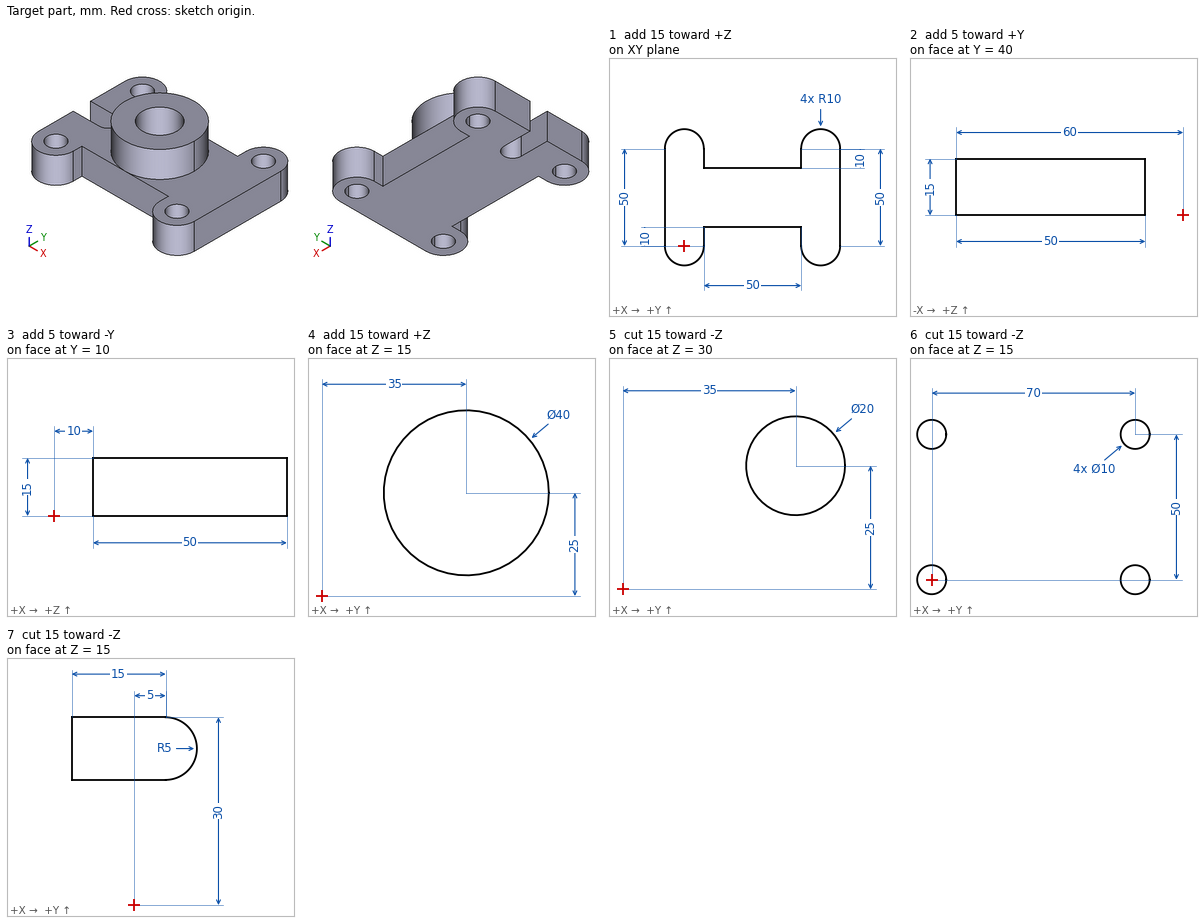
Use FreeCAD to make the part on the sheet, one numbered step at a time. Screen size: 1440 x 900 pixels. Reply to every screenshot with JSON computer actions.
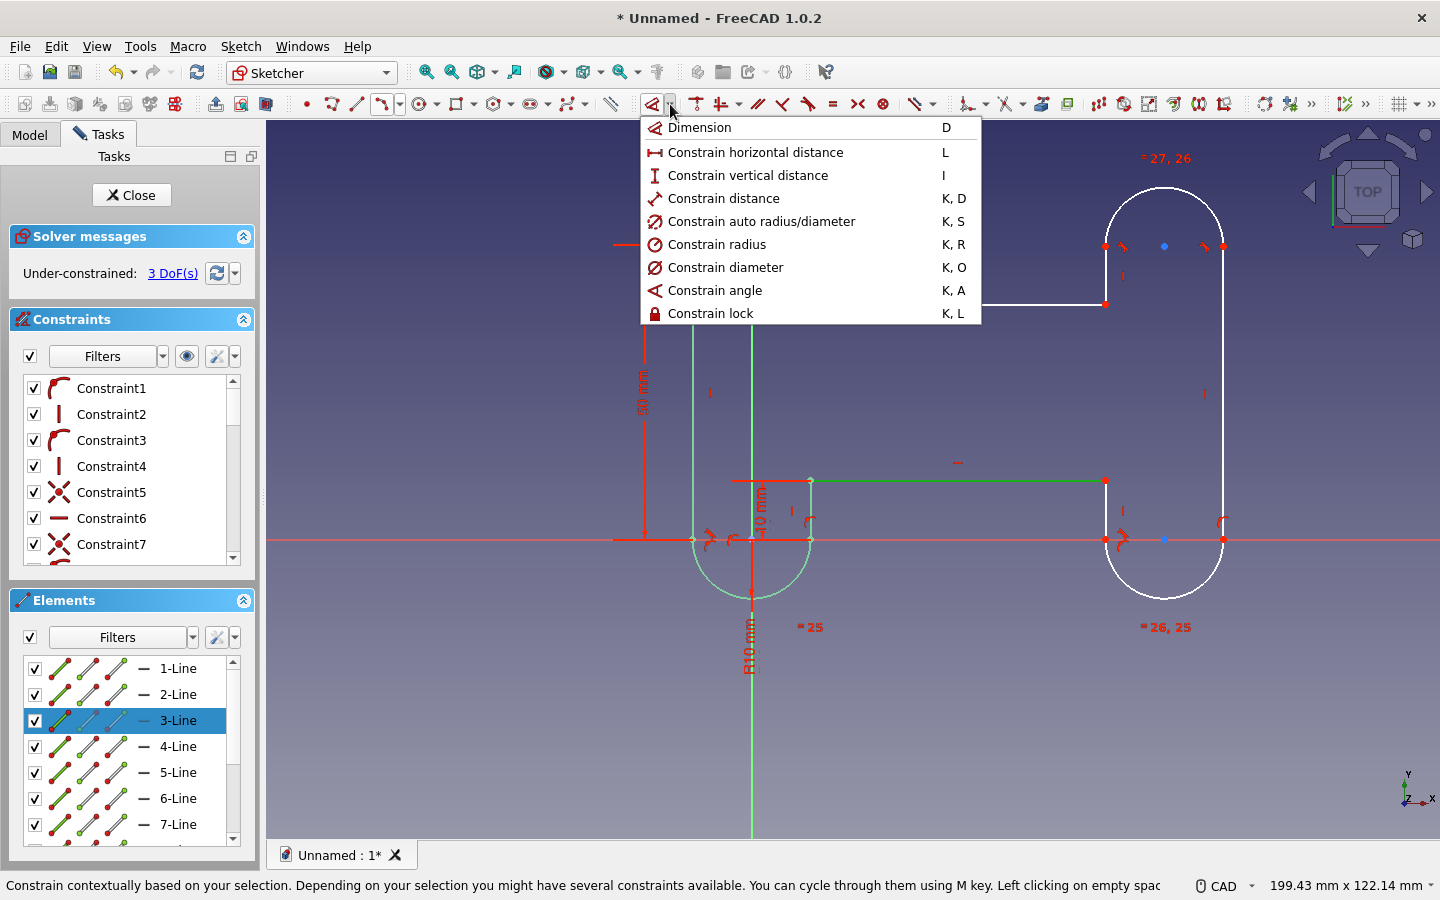
{"action": "left_click", "coordinate": [811, 152]}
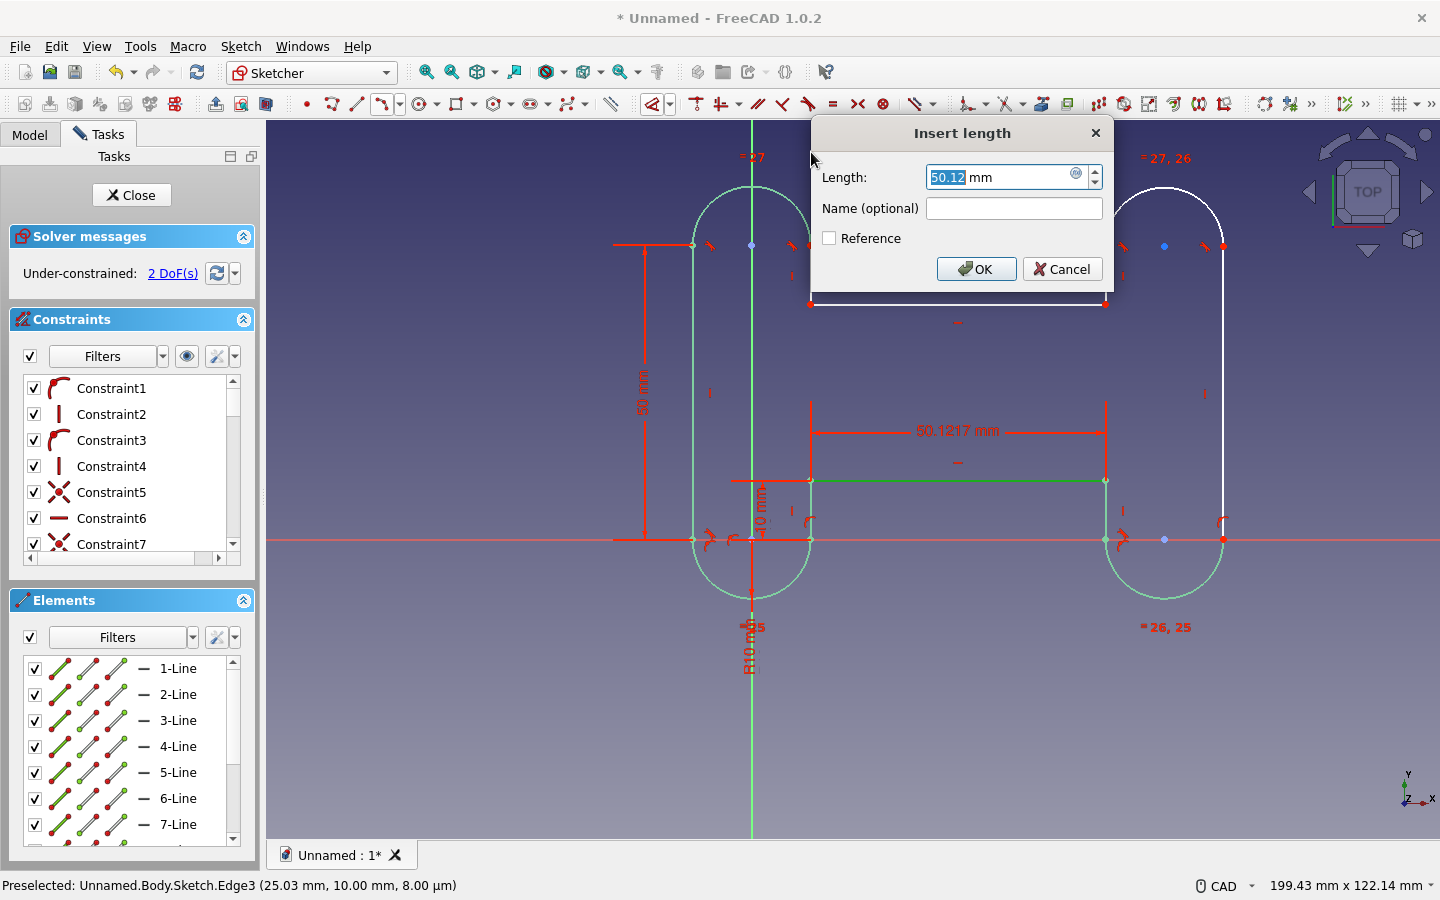
{"action": "type", "text": "50"}
{"action": "key", "text": "Return"}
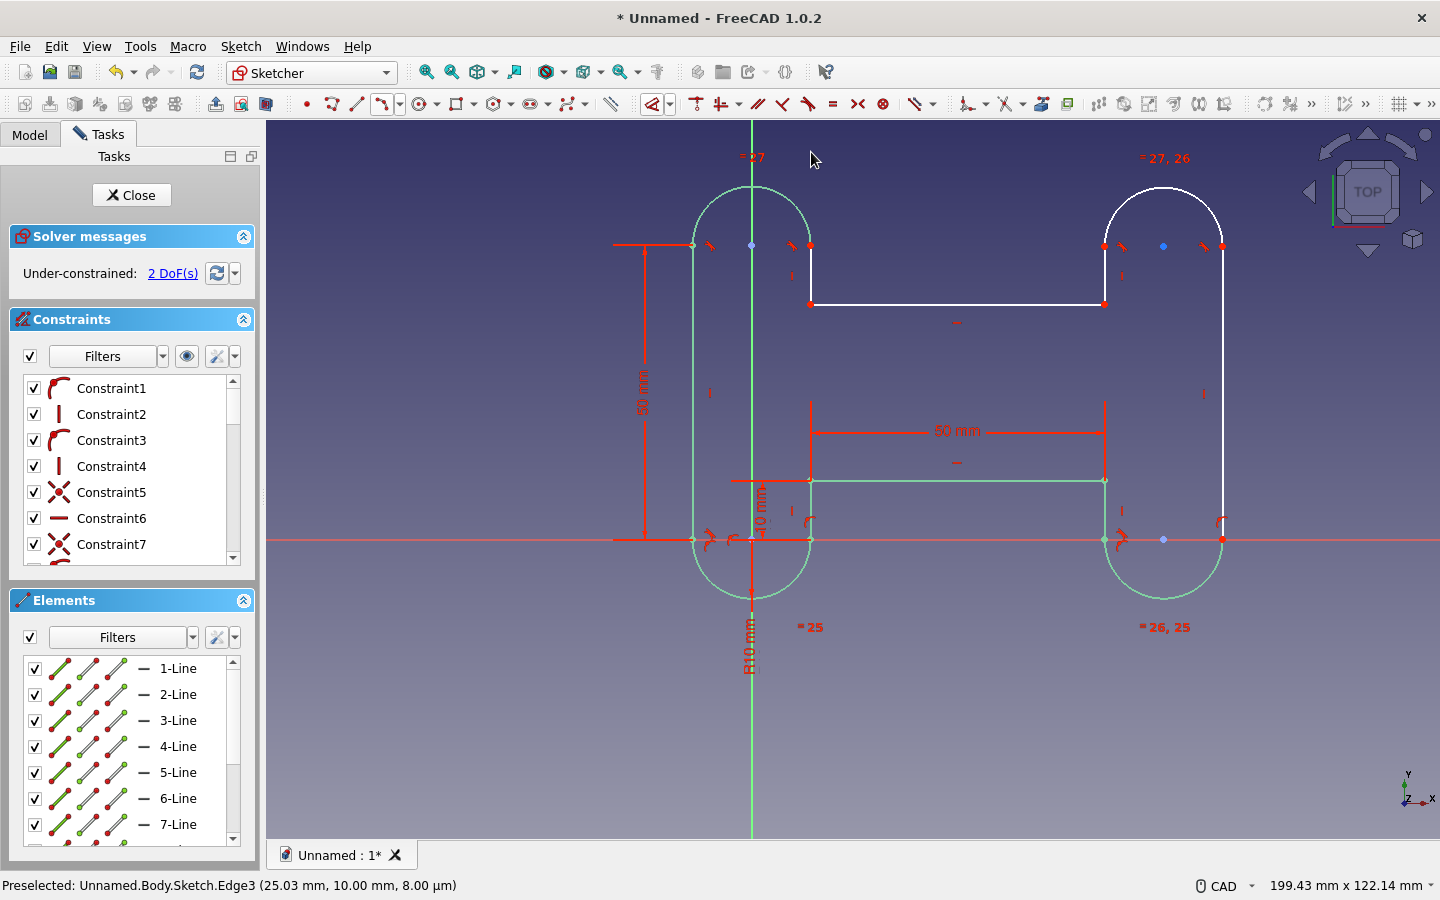
{"action": "left_click", "coordinate": [1223, 452]}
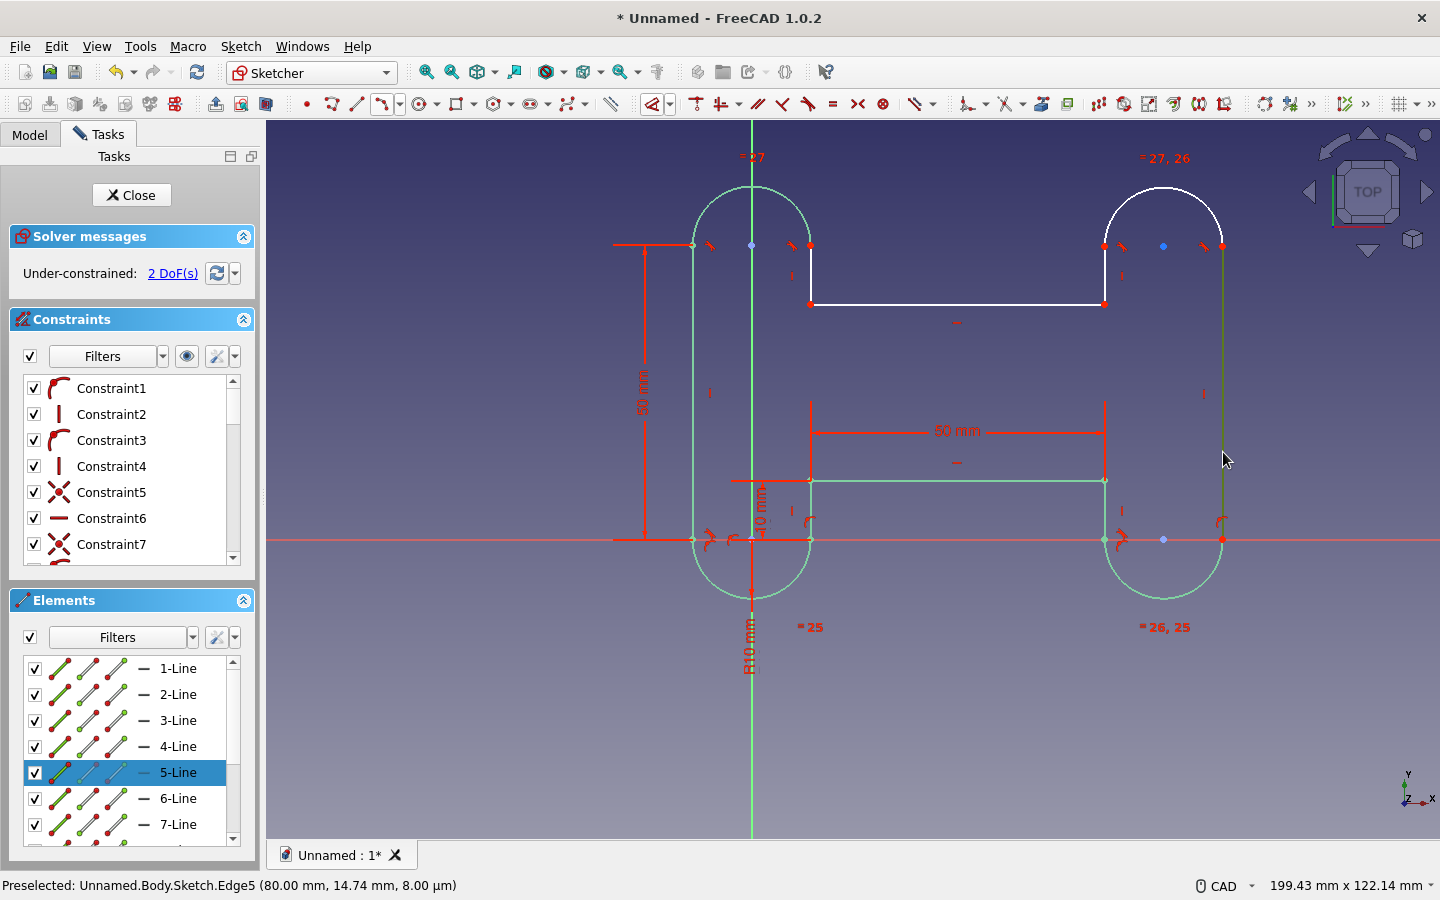
{"action": "left_click", "coordinate": [670, 104]}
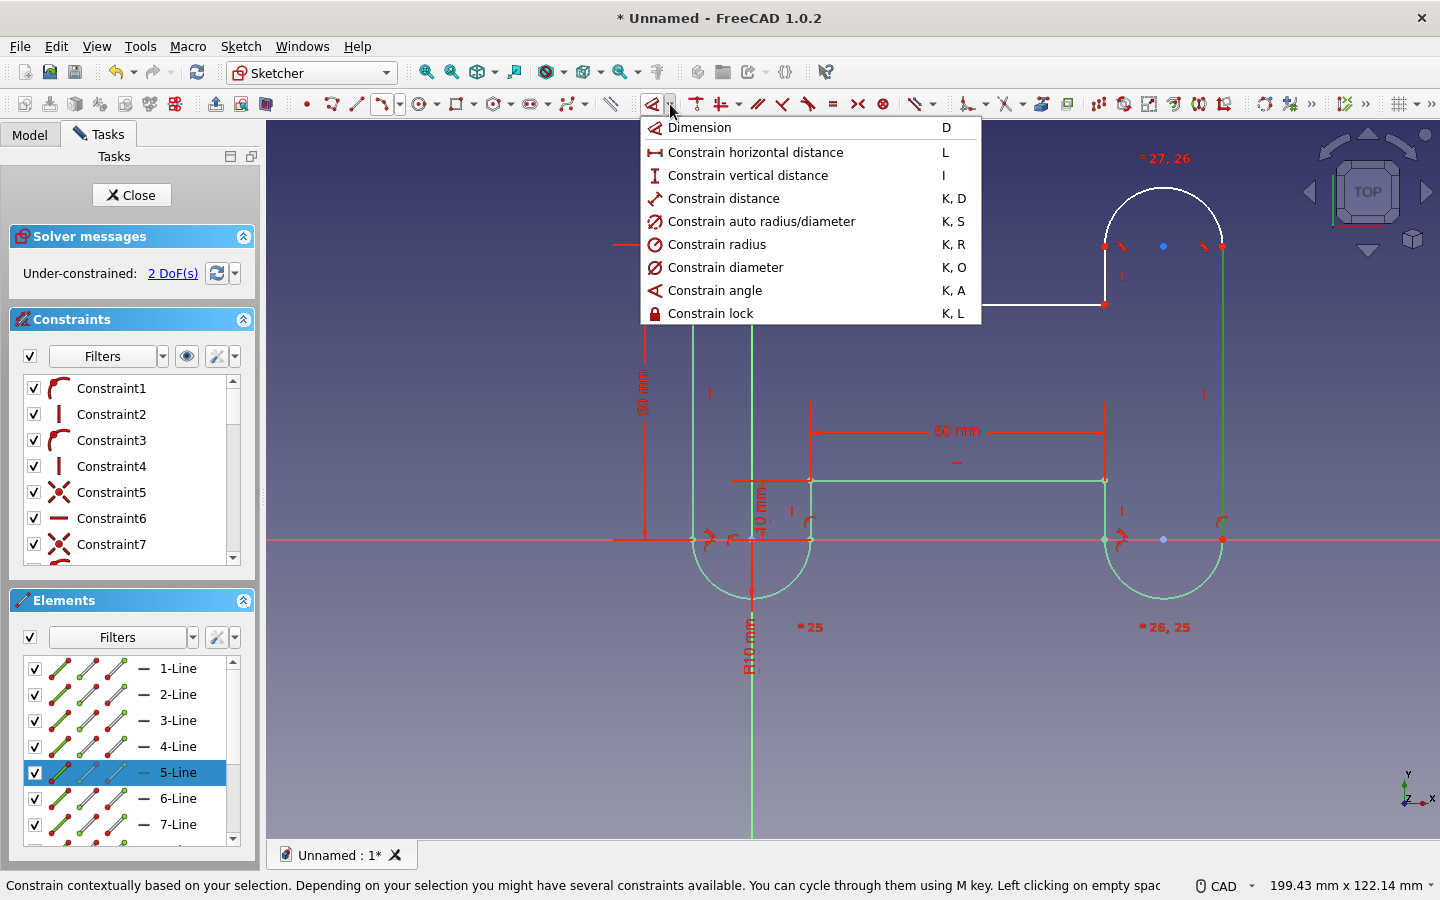
{"action": "left_click", "coordinate": [811, 176]}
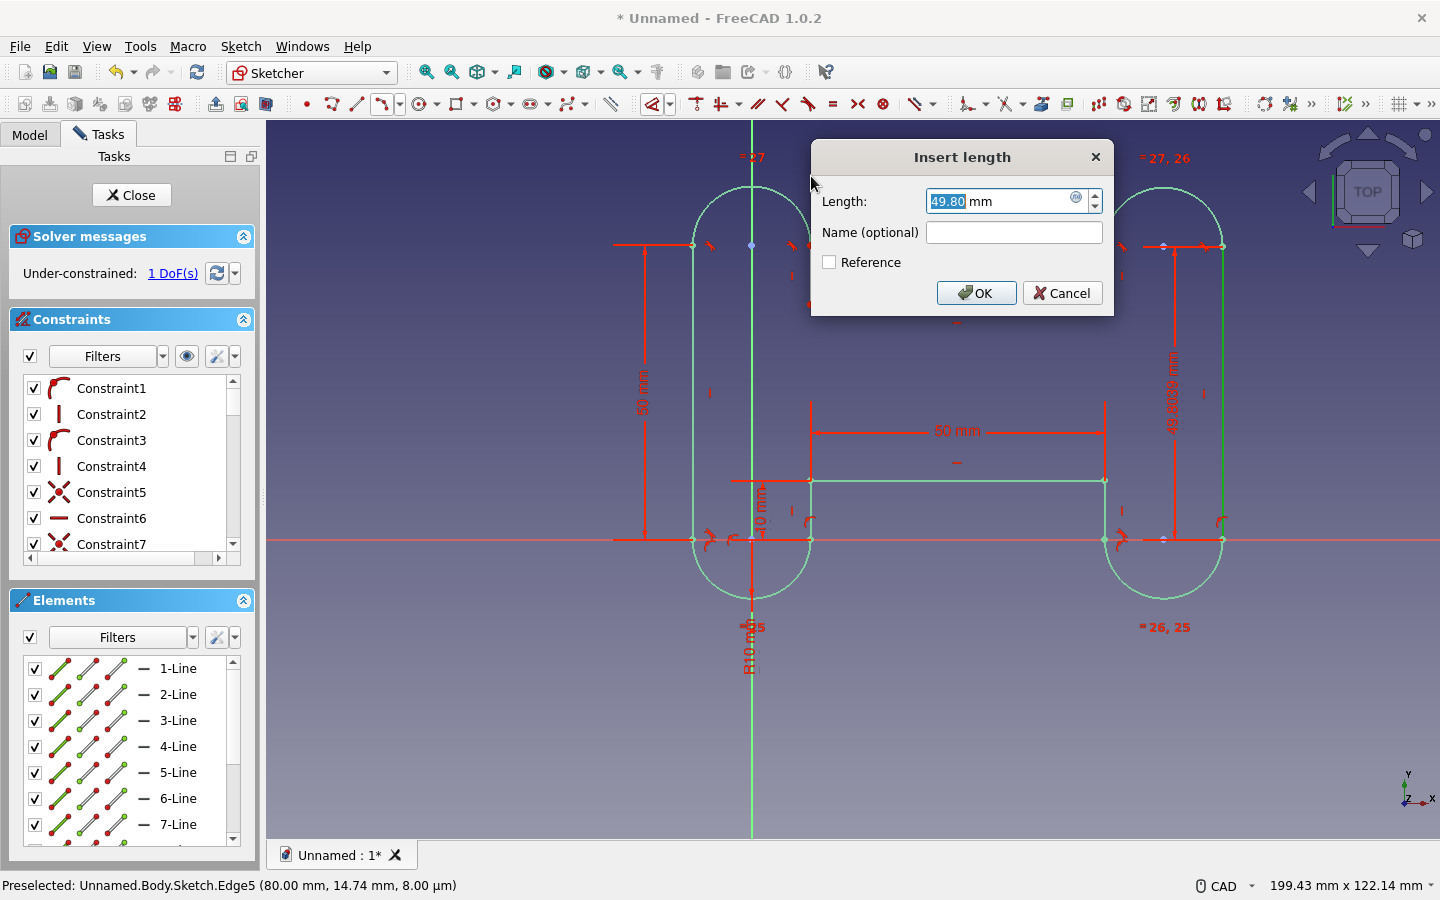
{"action": "type", "text": "50"}
{"action": "key", "text": "Return"}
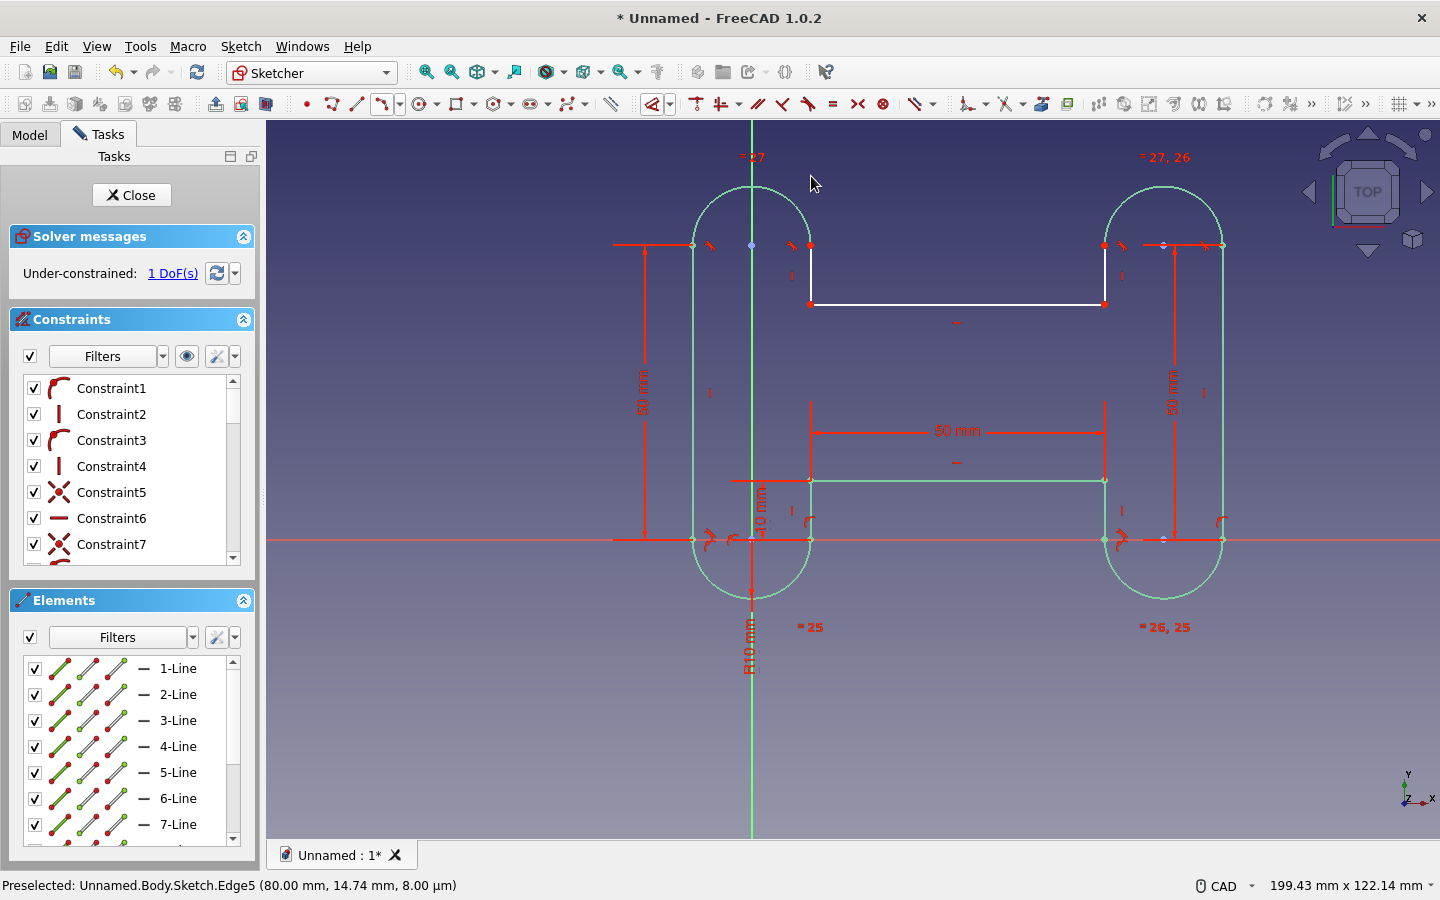
{"action": "left_click", "coordinate": [1105, 263]}